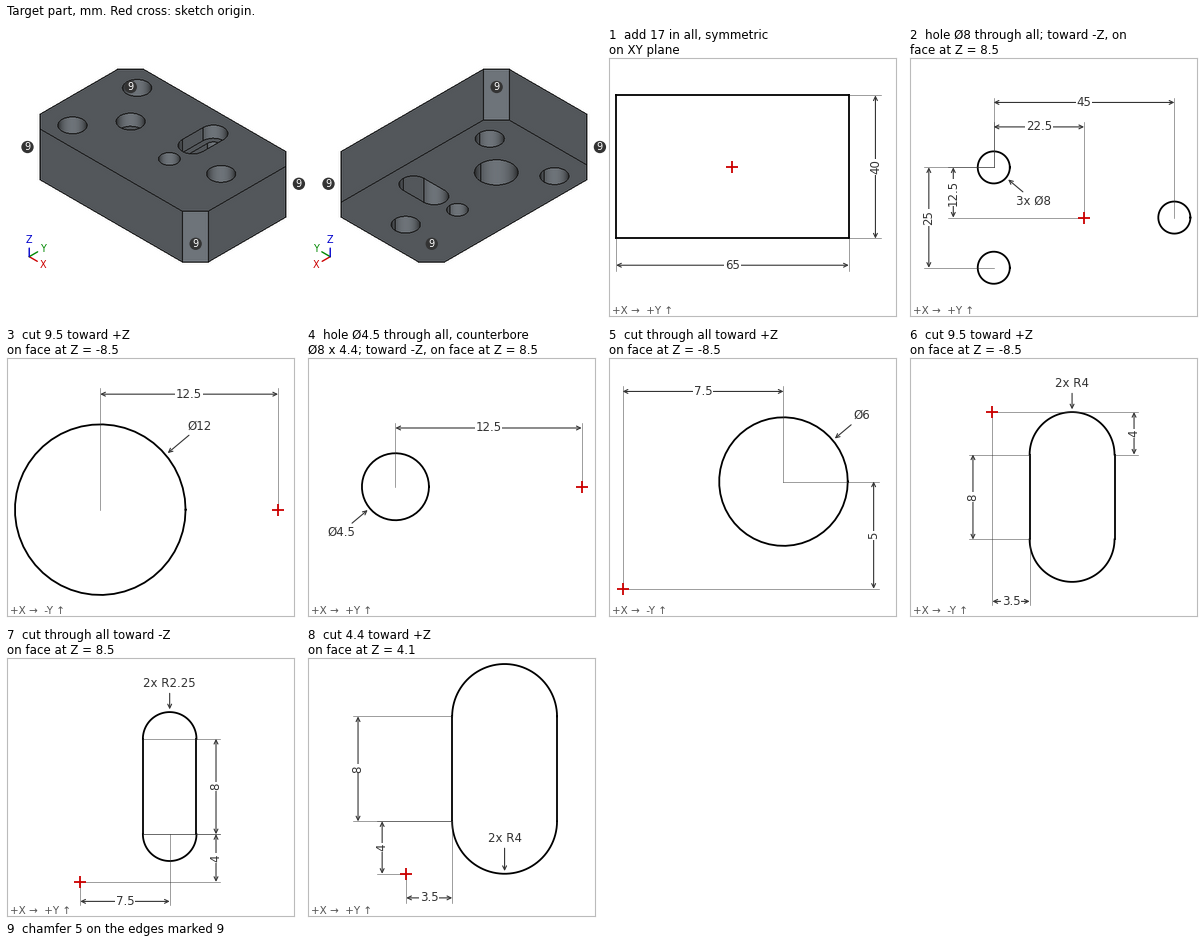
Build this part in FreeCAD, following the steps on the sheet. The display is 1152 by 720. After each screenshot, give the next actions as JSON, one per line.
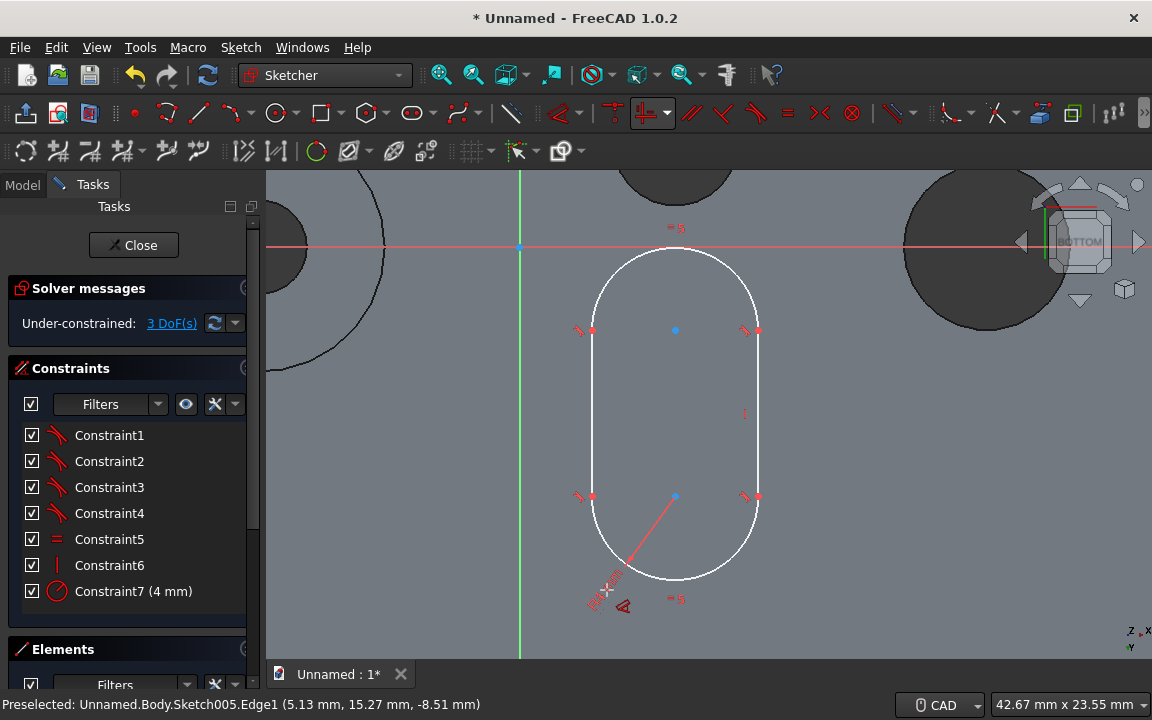
{"action": "left_click", "coordinate": [592, 447]}
{"action": "left_click", "coordinate": [558, 414]}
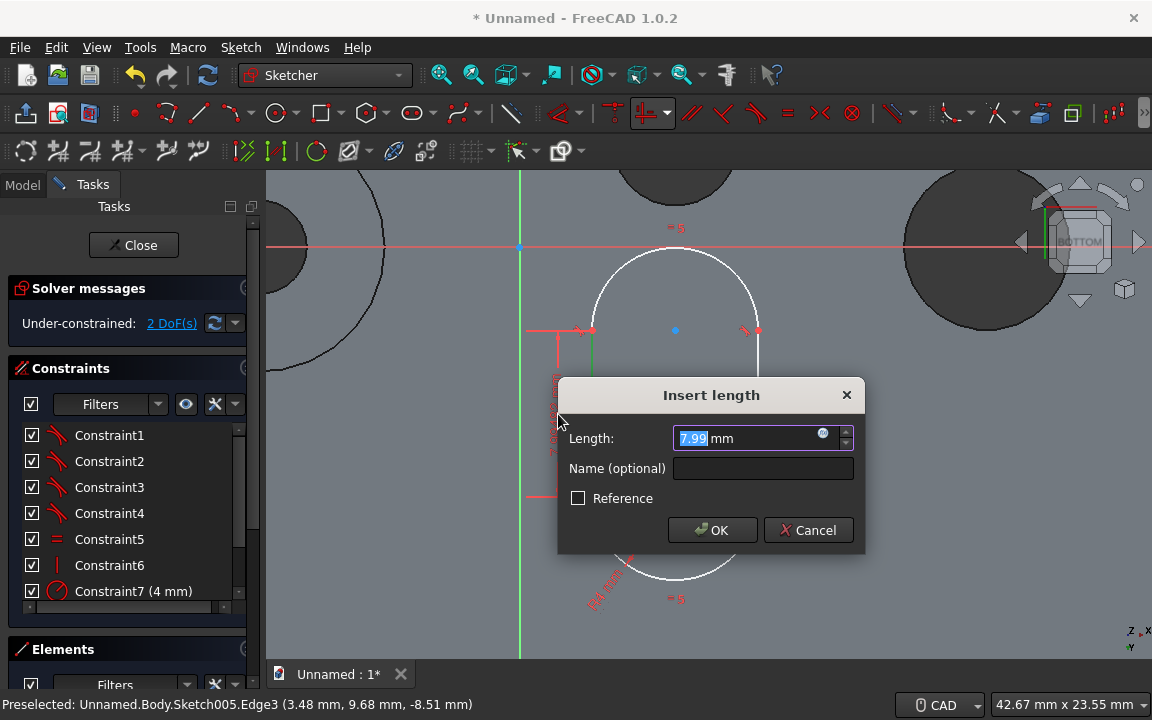
{"action": "type", "text": "8"}
{"action": "key", "text": "Return"}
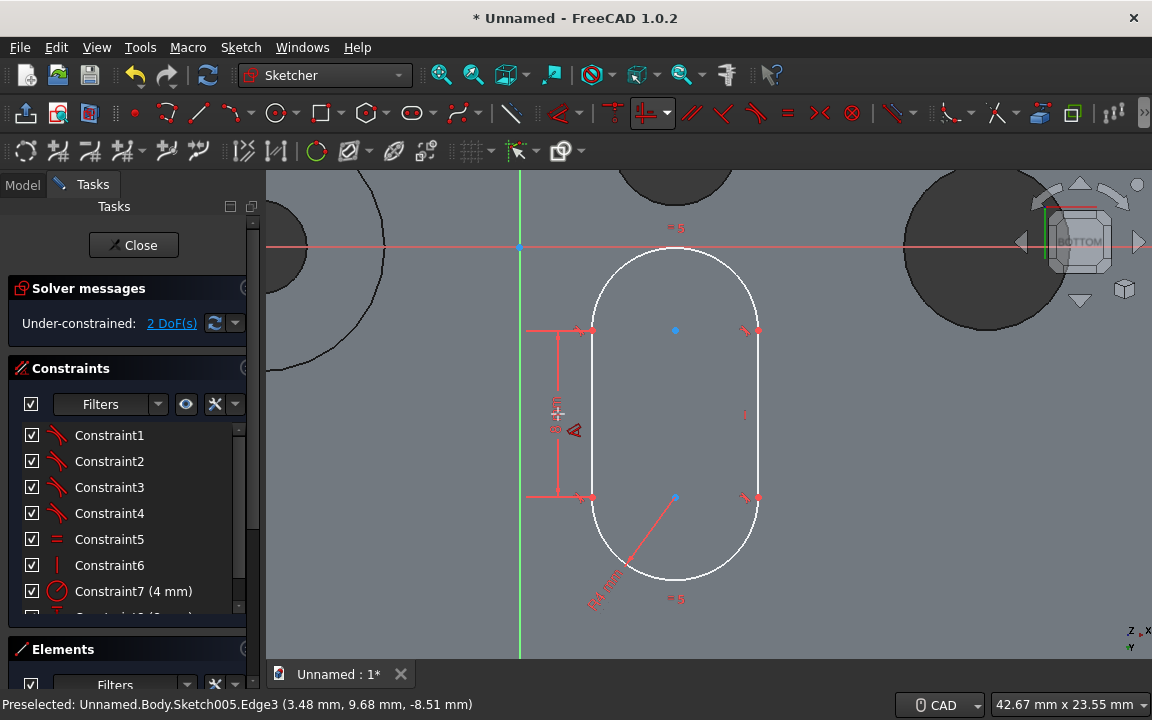
{"action": "left_click", "coordinate": [758, 331]}
{"action": "left_click", "coordinate": [486, 289]}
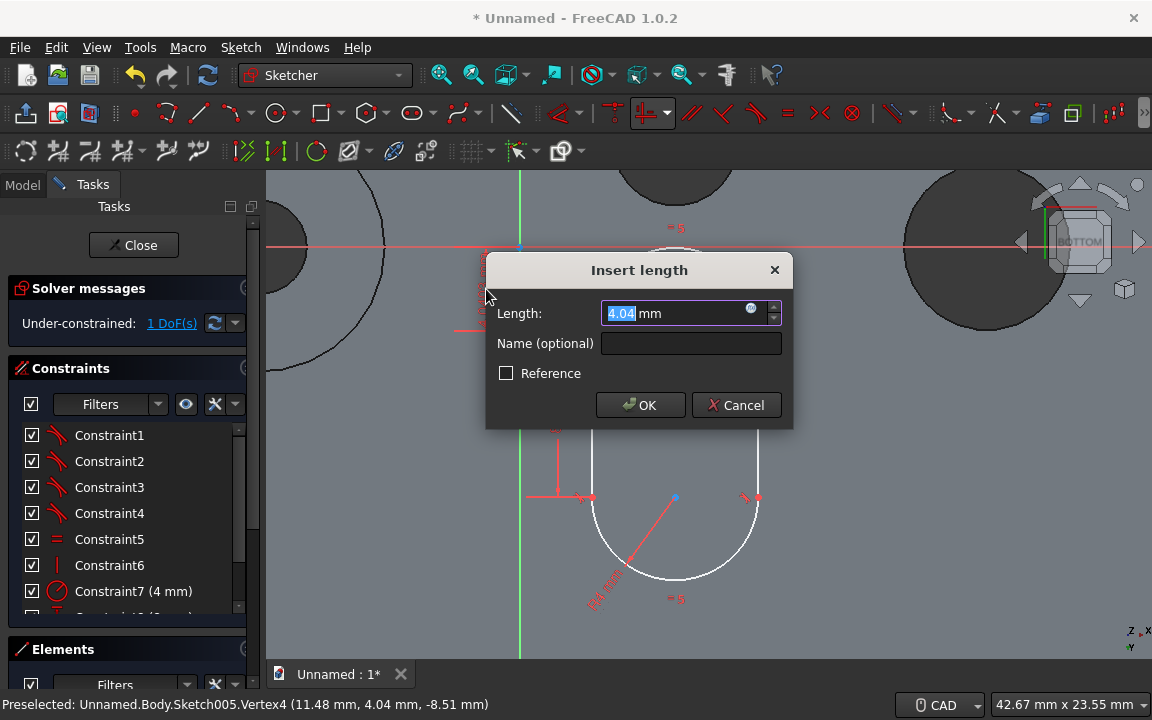
{"action": "type", "text": "4"}
{"action": "key", "text": "Return"}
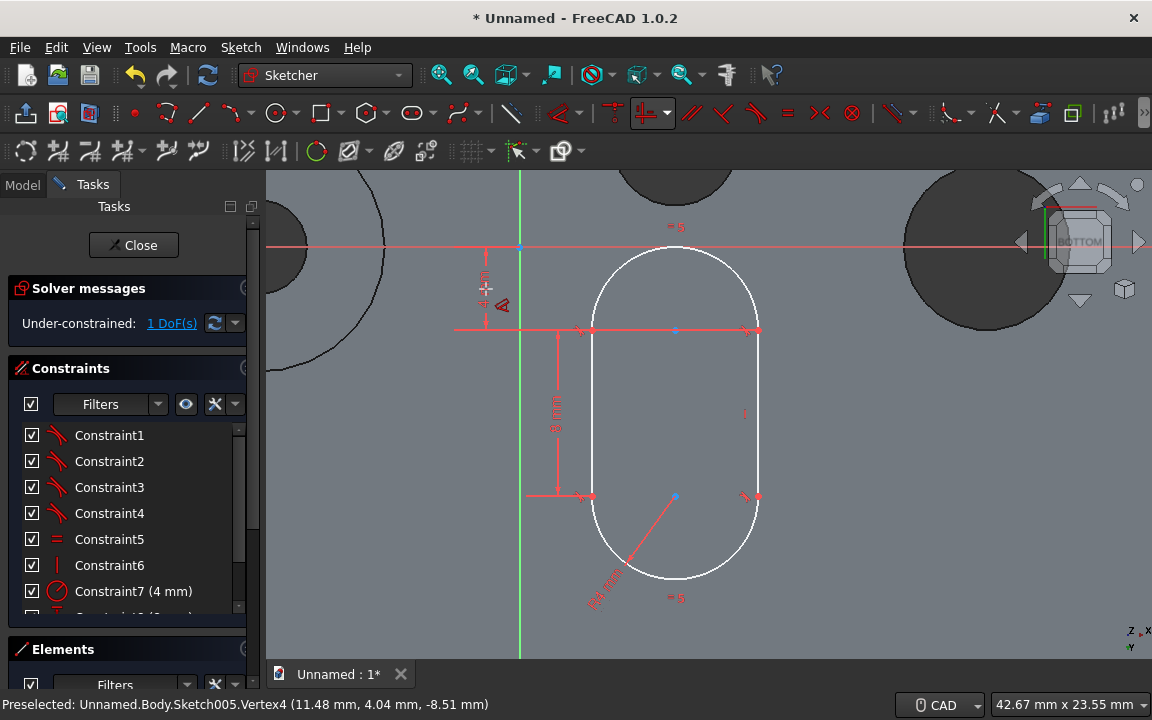
{"action": "left_click", "coordinate": [592, 496]}
{"action": "left_click", "coordinate": [556, 213]}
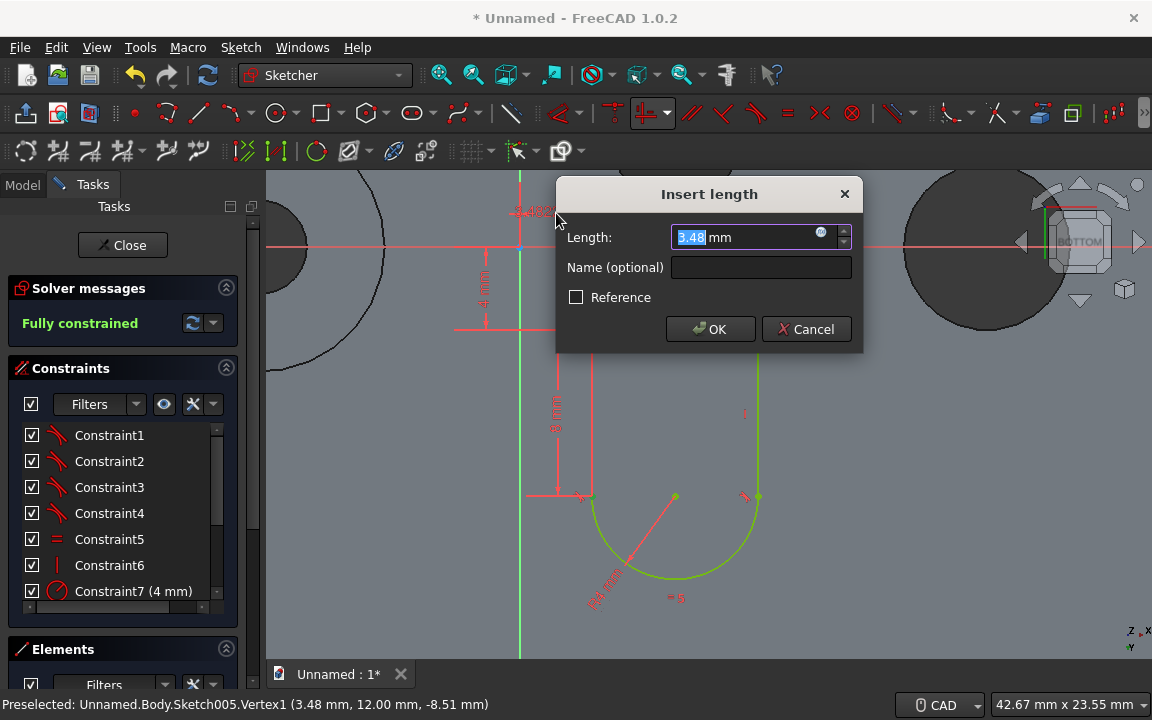
{"action": "type", "text": "3.5"}
{"action": "key", "text": "Return"}
{"action": "key", "text": "Escape"}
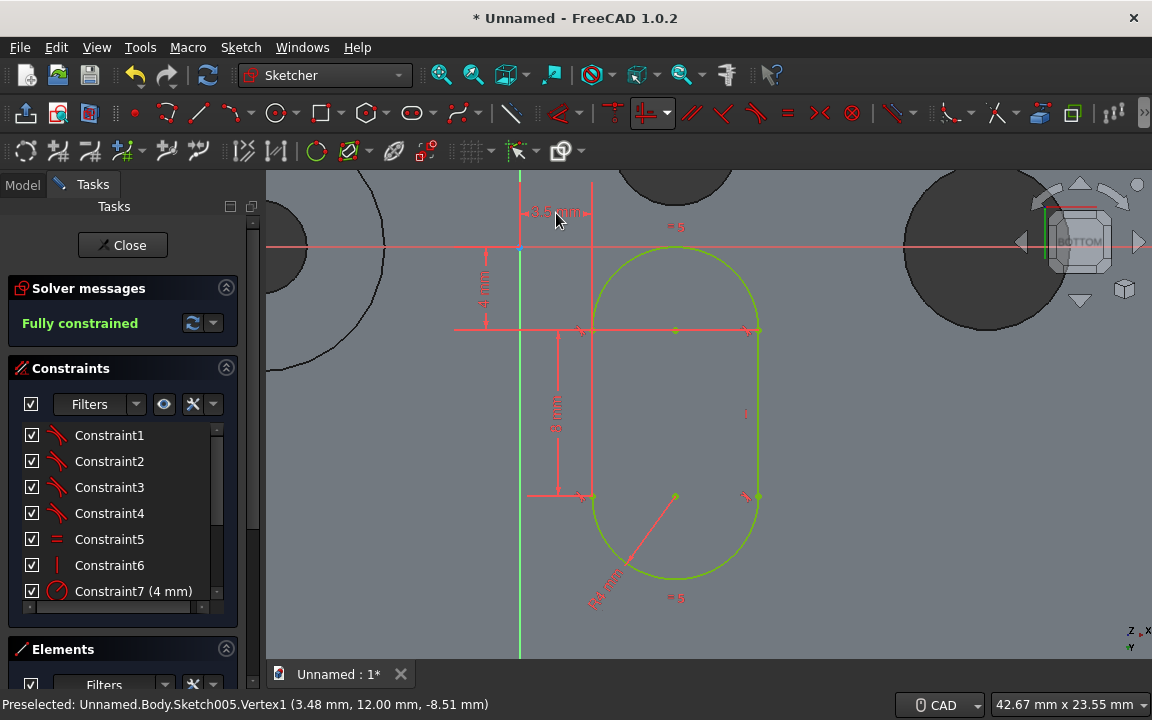
{"action": "left_click", "coordinate": [123, 245]}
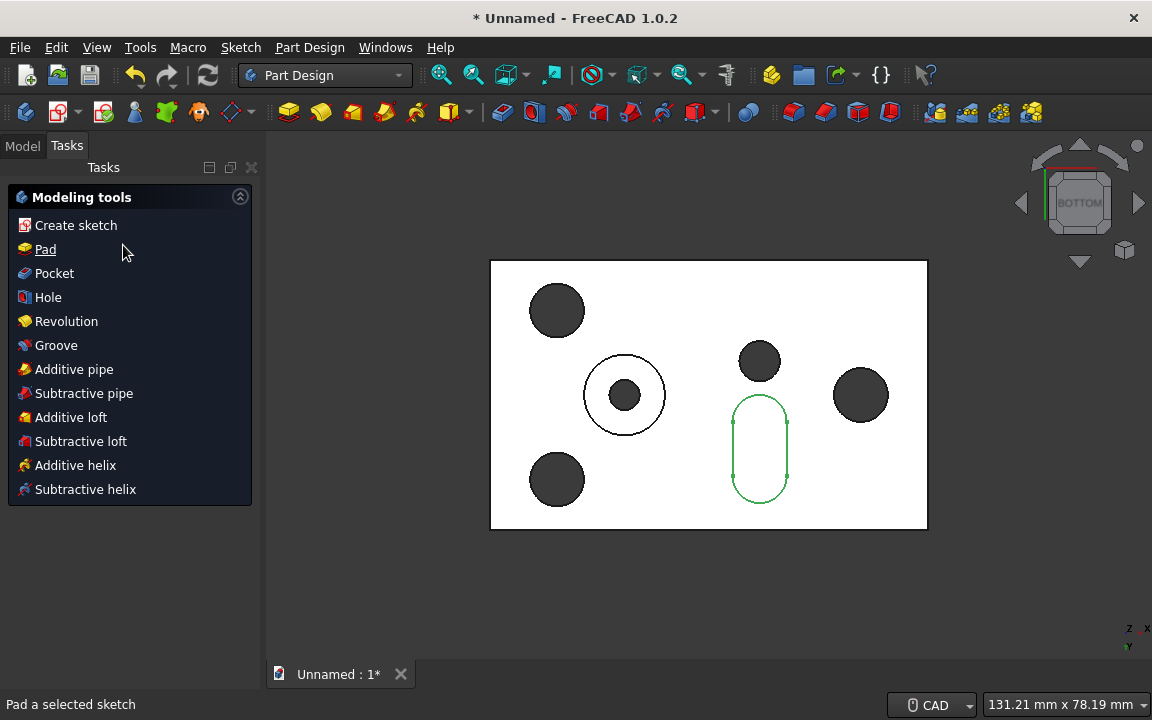
{"action": "left_click", "coordinate": [504, 112]}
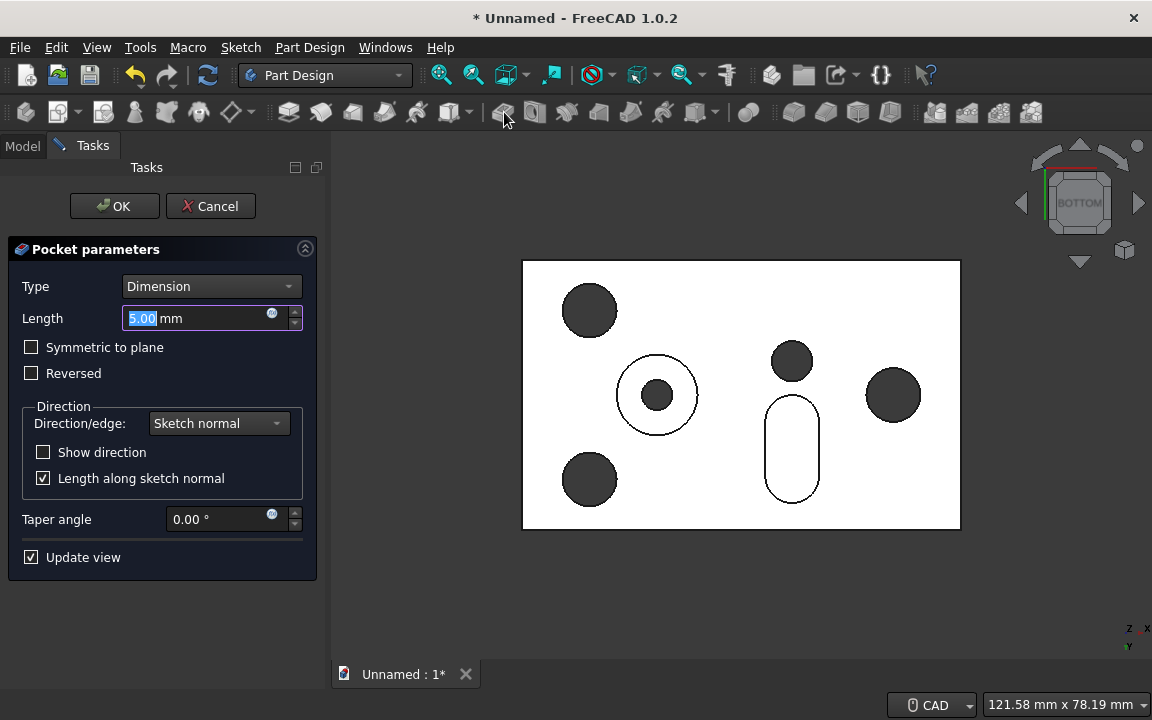
{"action": "type", "text": "9.5"}
{"action": "key", "text": "Tab"}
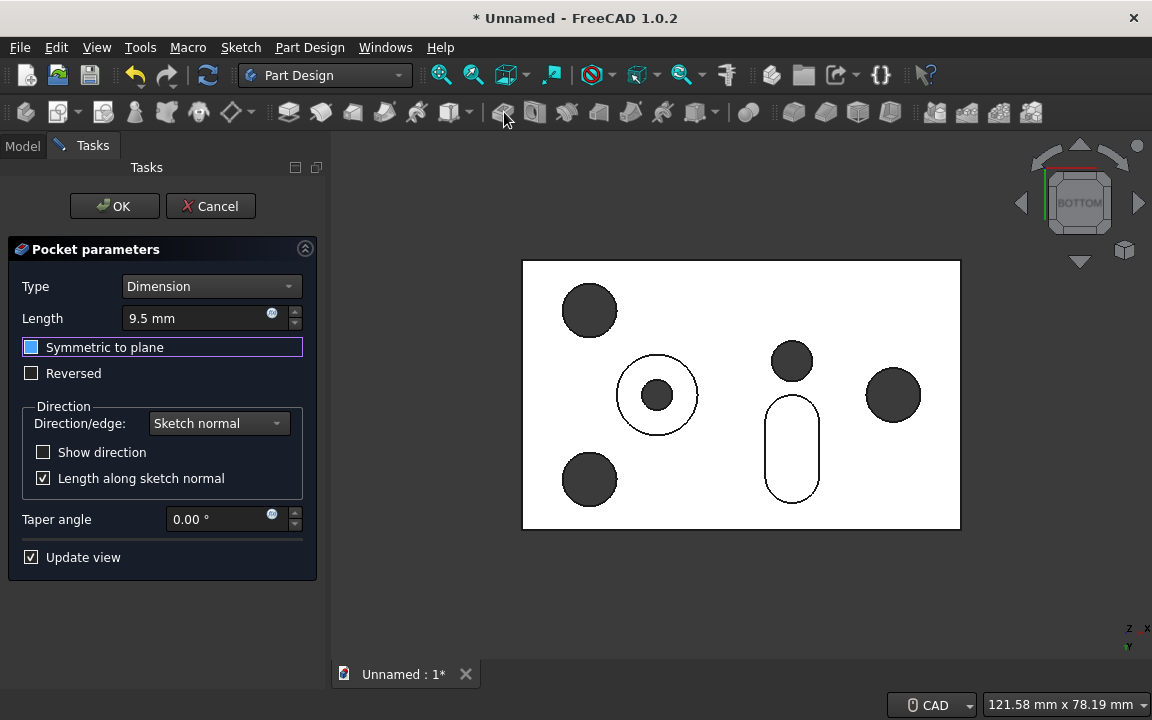
{"action": "left_click", "coordinate": [115, 206]}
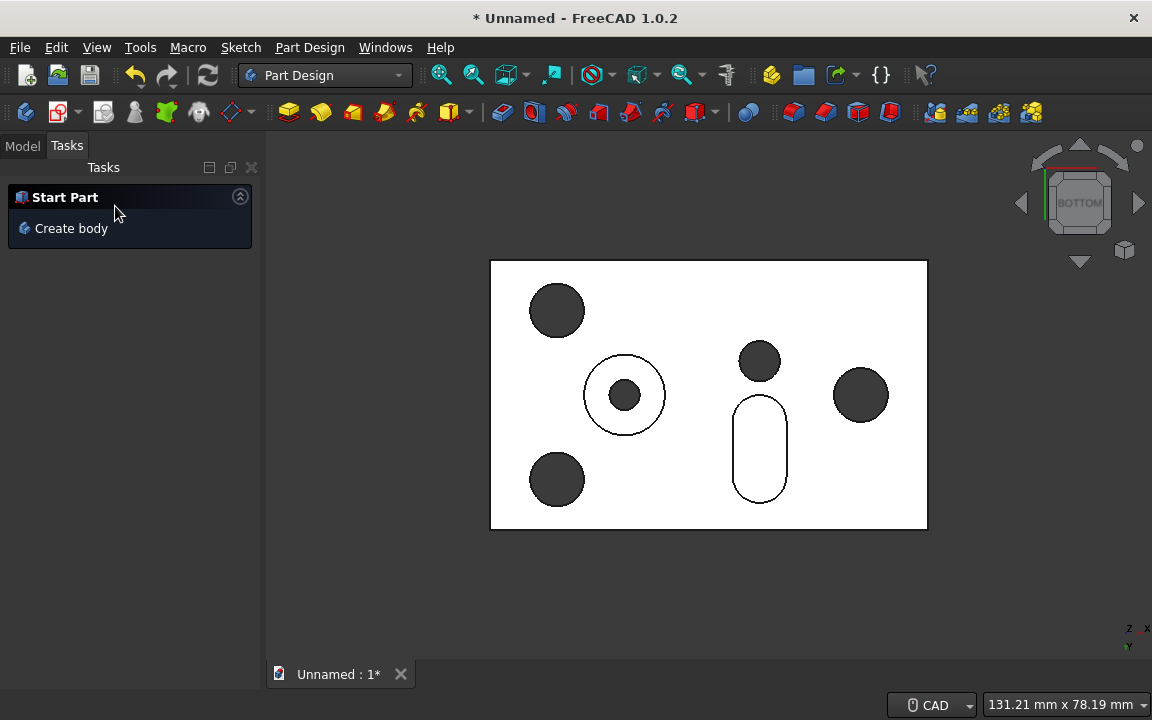
{"action": "key", "text": "0"}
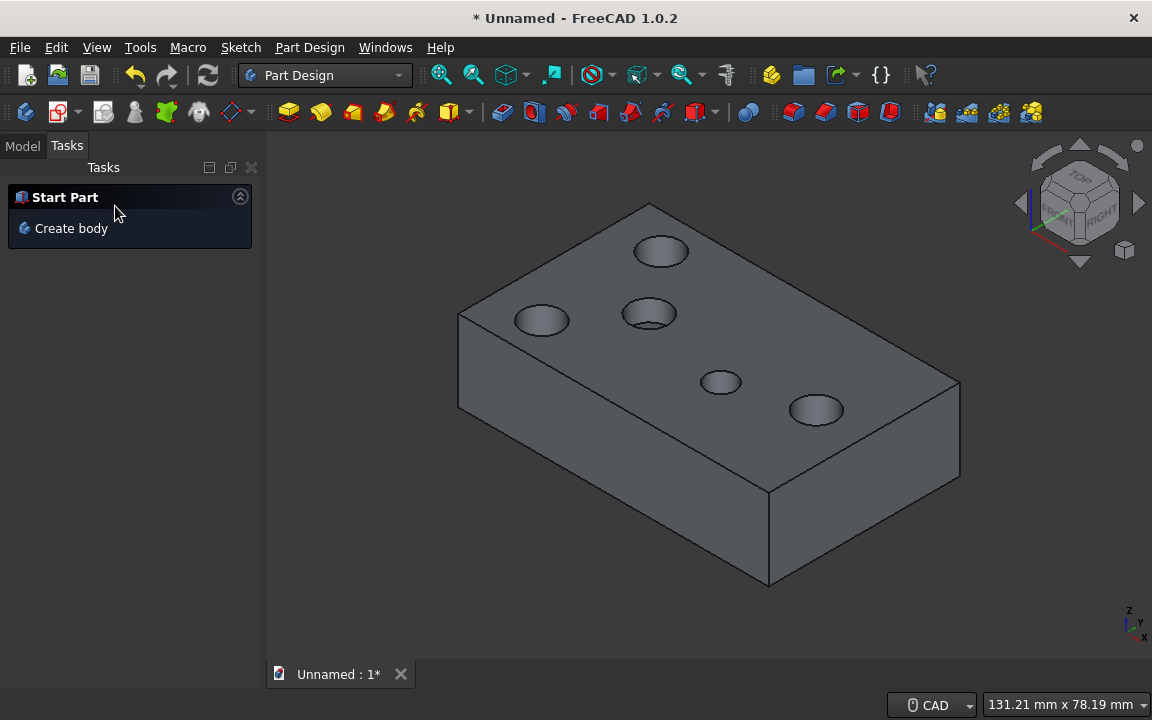
{"action": "left_click", "coordinate": [736, 331]}